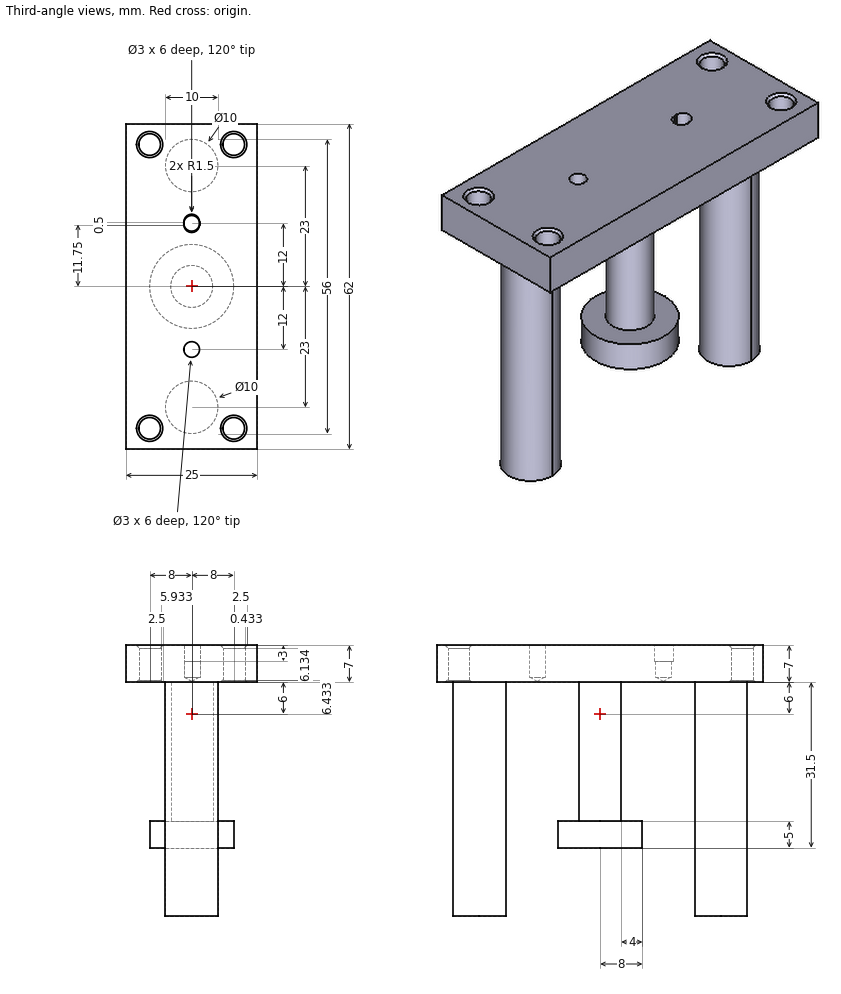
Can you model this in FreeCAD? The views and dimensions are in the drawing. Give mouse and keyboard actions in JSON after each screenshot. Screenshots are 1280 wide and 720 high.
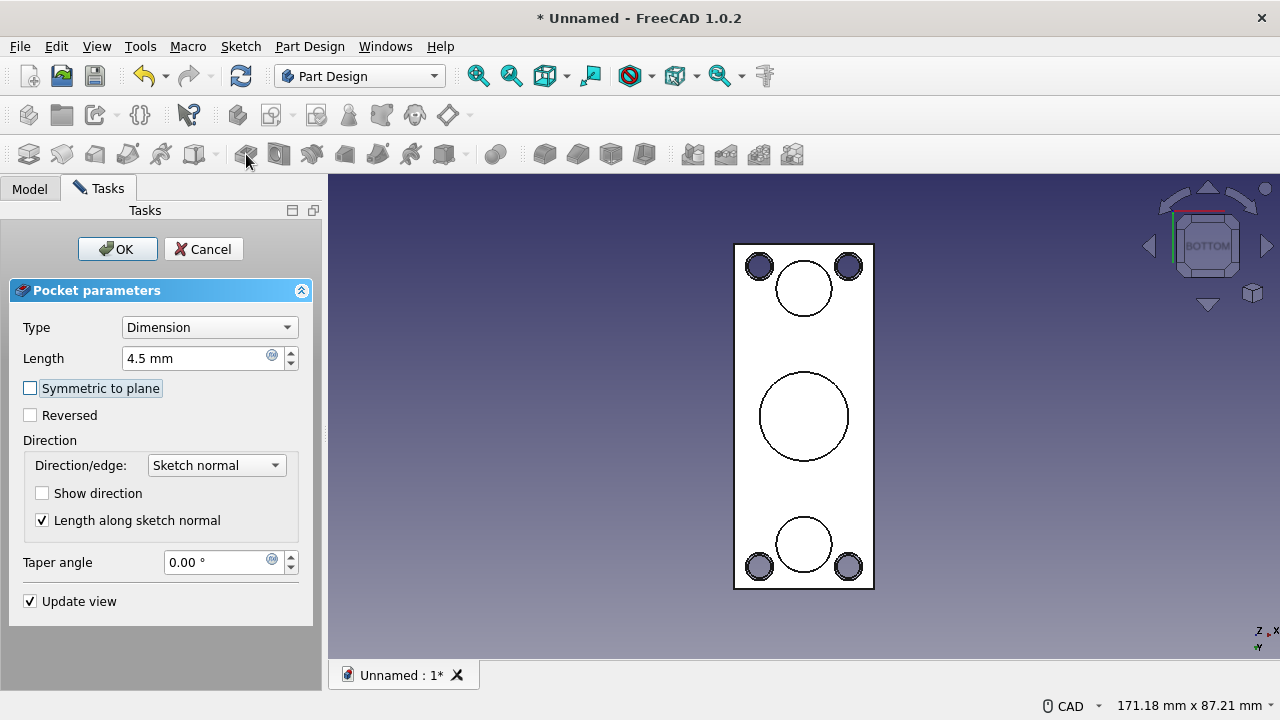
{"action": "left_click", "coordinate": [118, 249]}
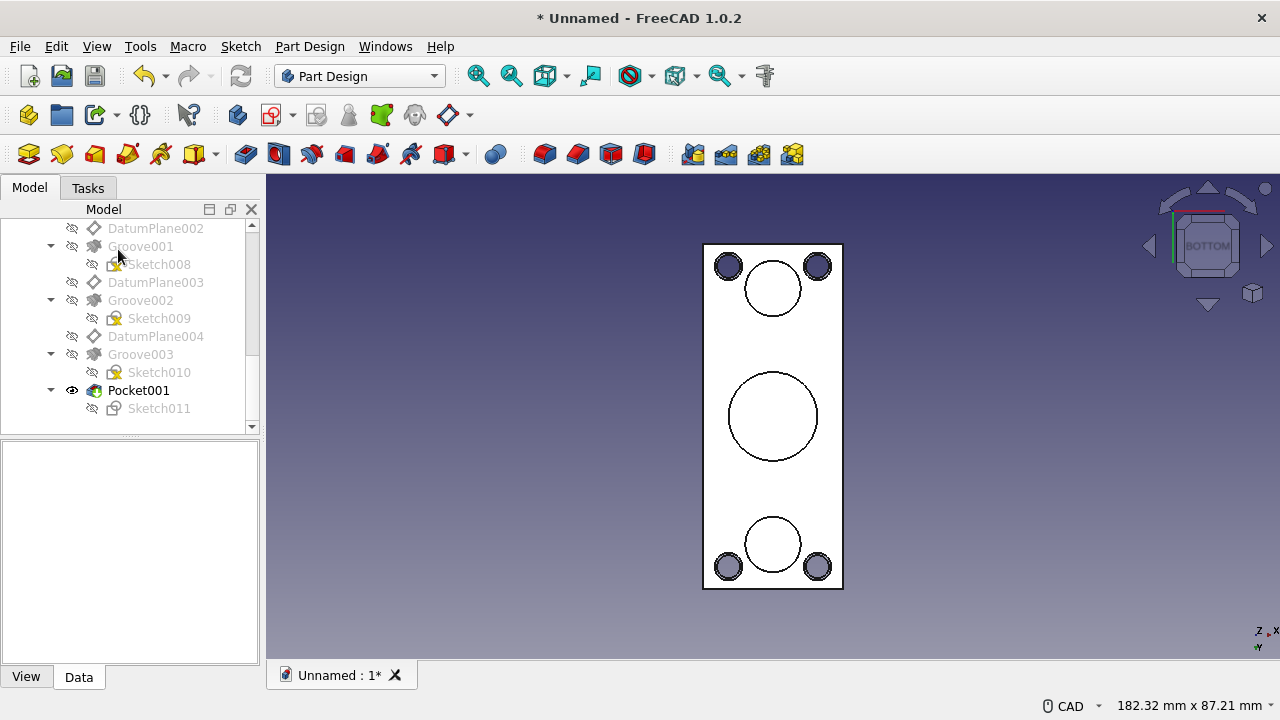
{"action": "key", "text": "0"}